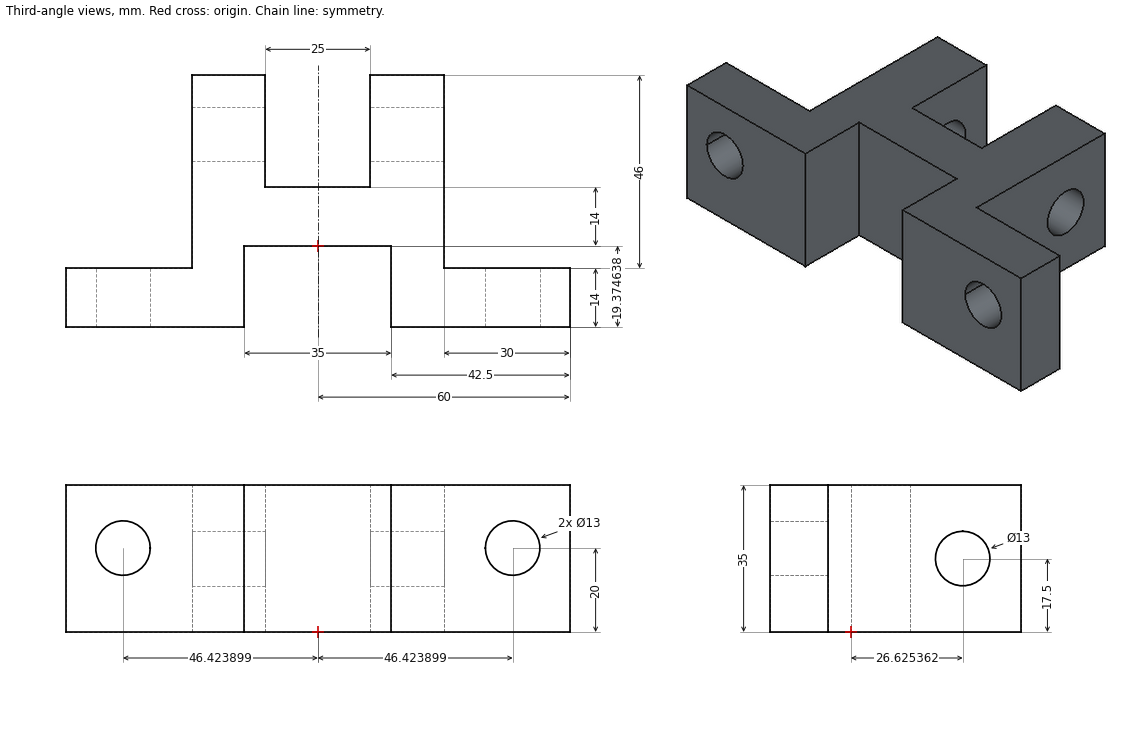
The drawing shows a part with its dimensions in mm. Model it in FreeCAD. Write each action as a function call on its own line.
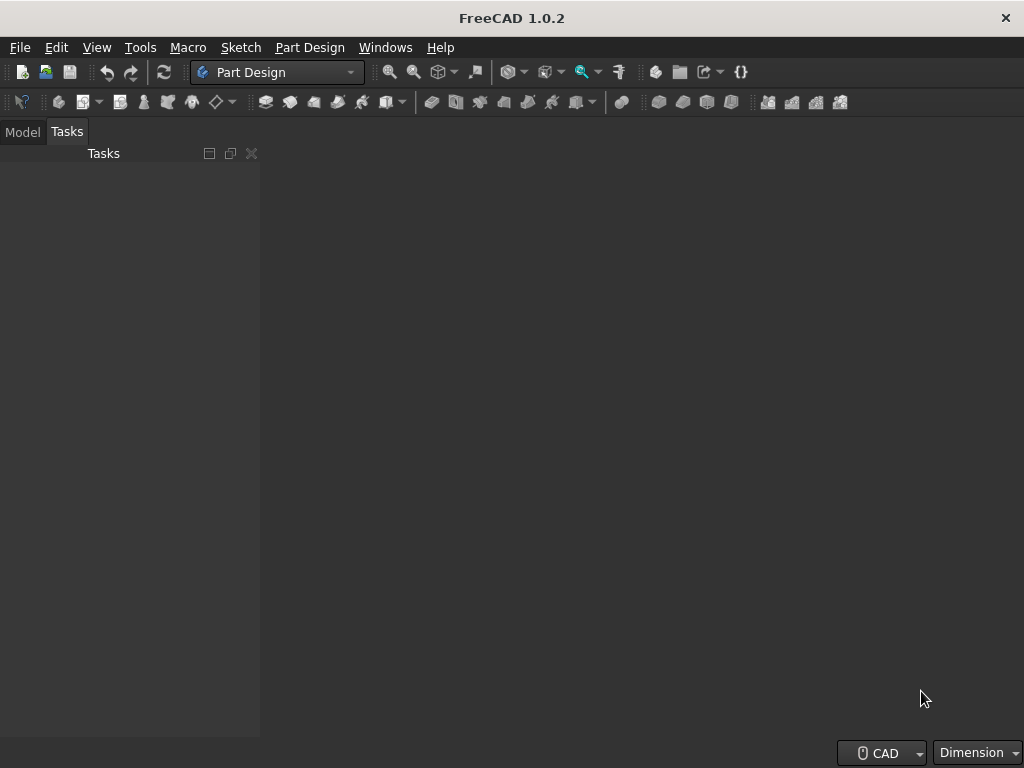
click(22, 72)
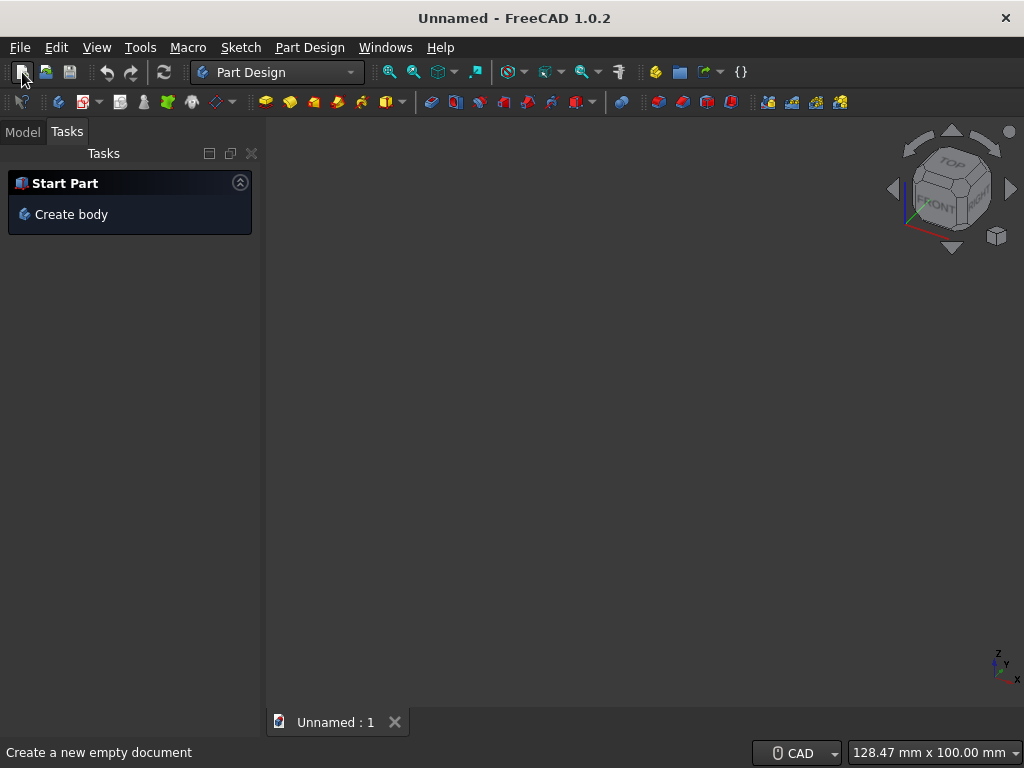
click(84, 102)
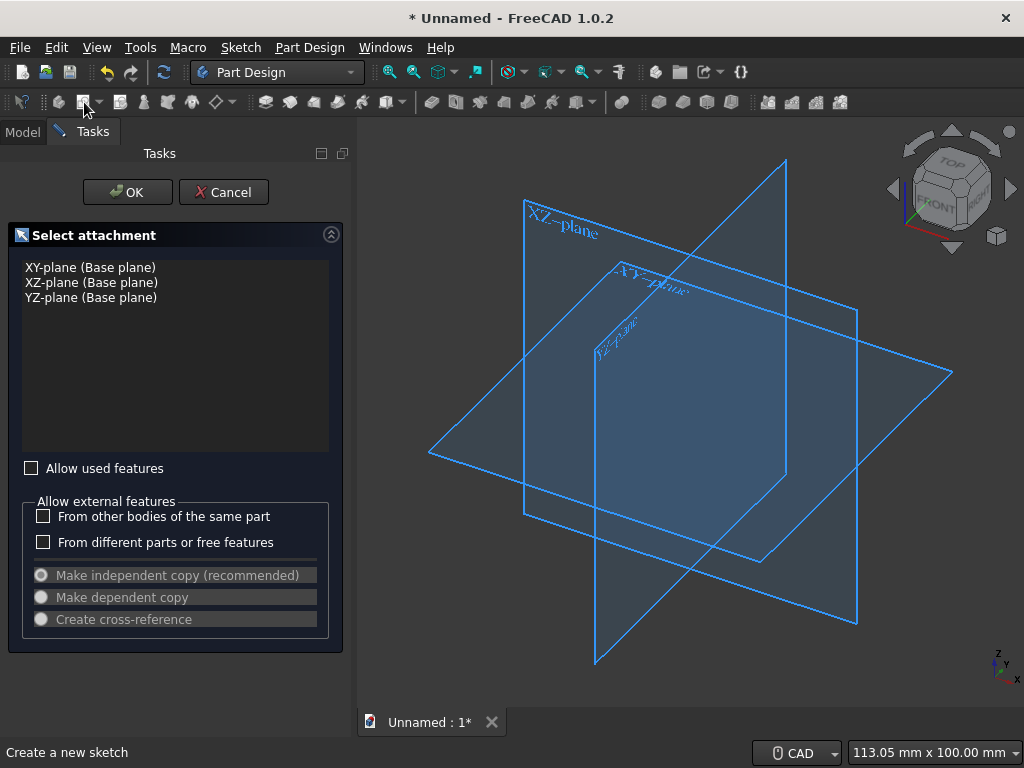
click(82, 268)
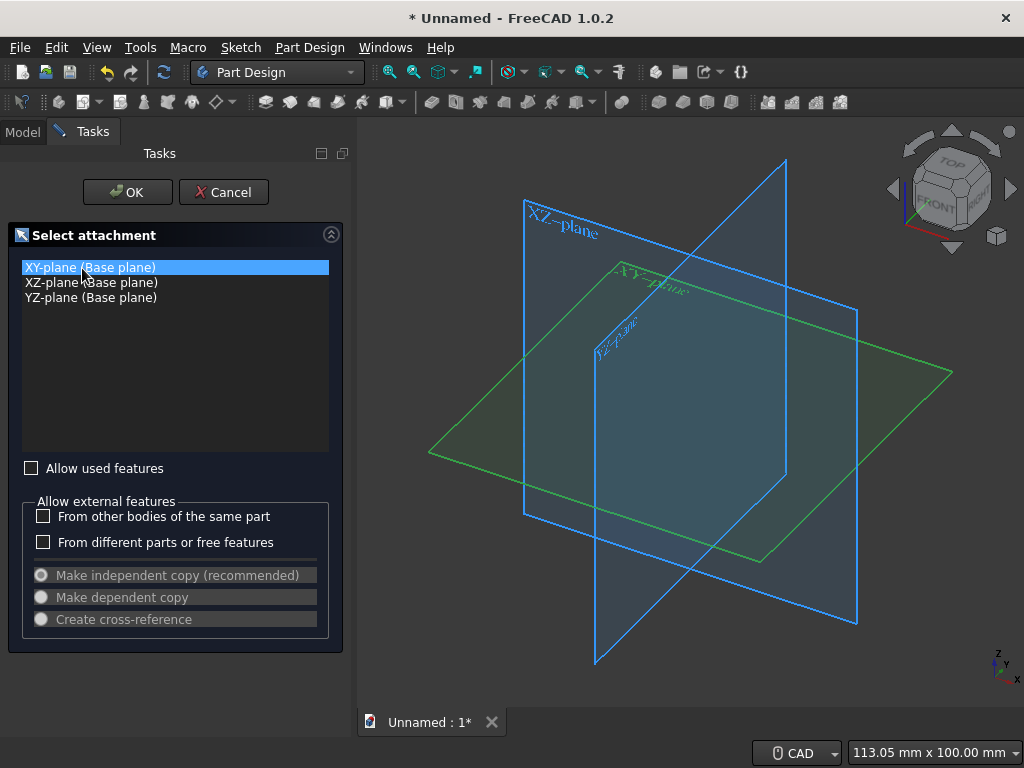
click(128, 192)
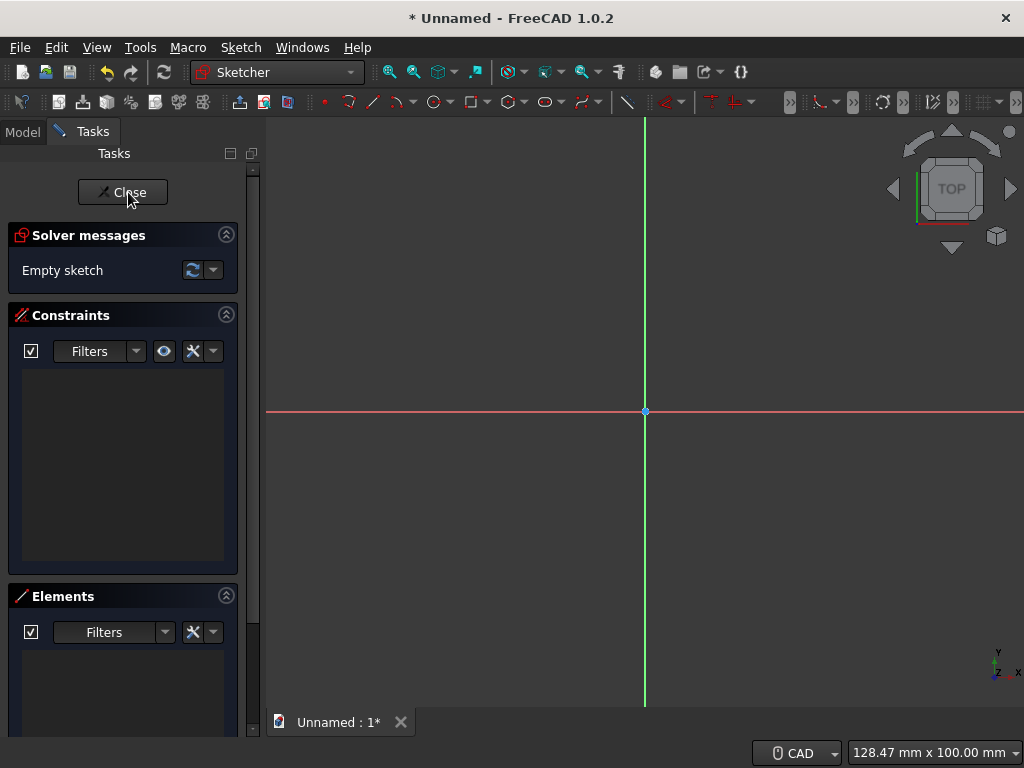
scroll(493, 488, down, 3)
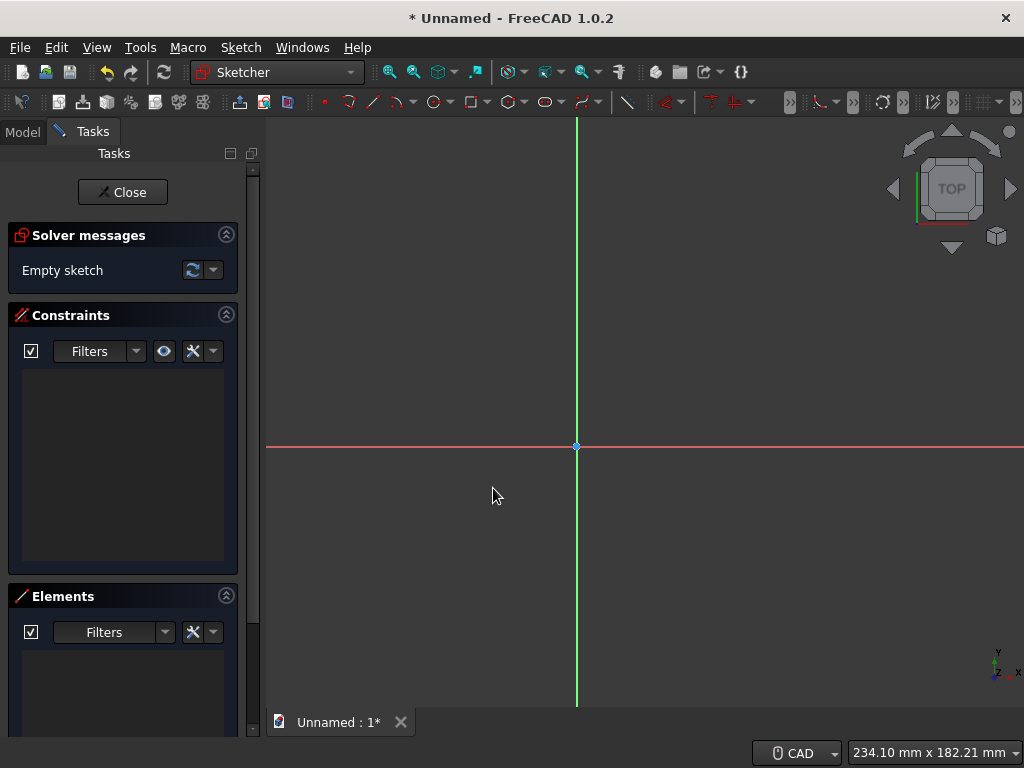
click(350, 102)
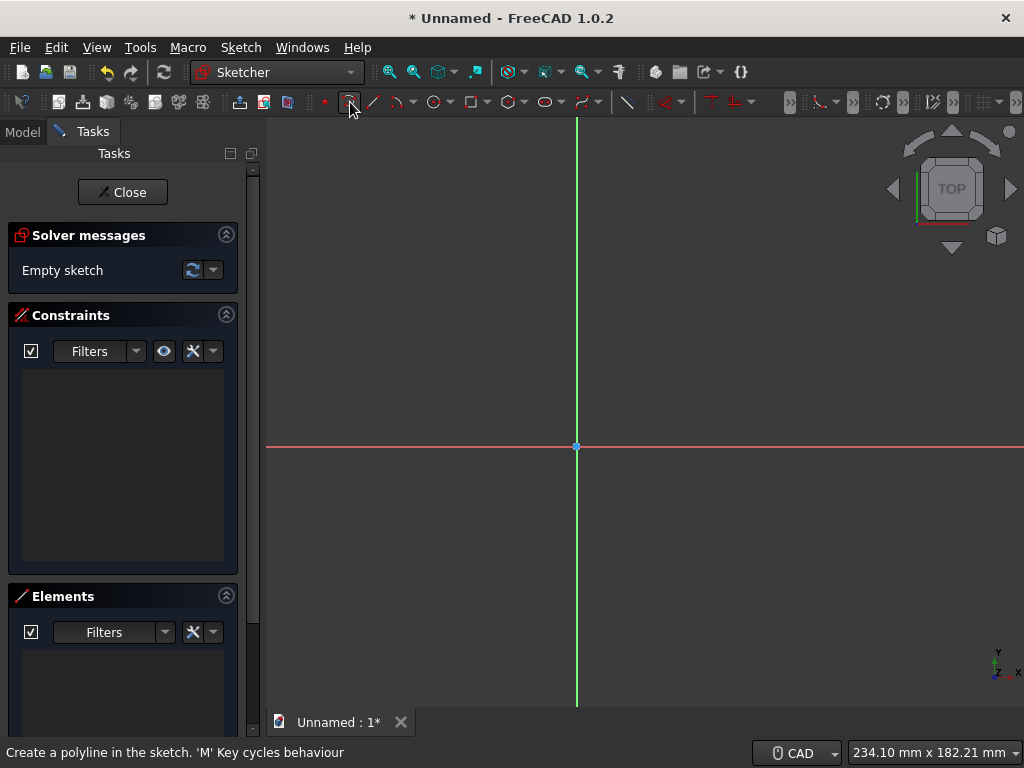
click(633, 447)
click(633, 509)
click(771, 509)
click(771, 464)
click(674, 464)
click(674, 315)
click(617, 315)
click(617, 401)
click(536, 401)
click(536, 315)
click(479, 315)
click(479, 464)
click(382, 464)
click(382, 509)
click(520, 509)
click(520, 438)
click(633, 447)
key(Escape)
key(Escape)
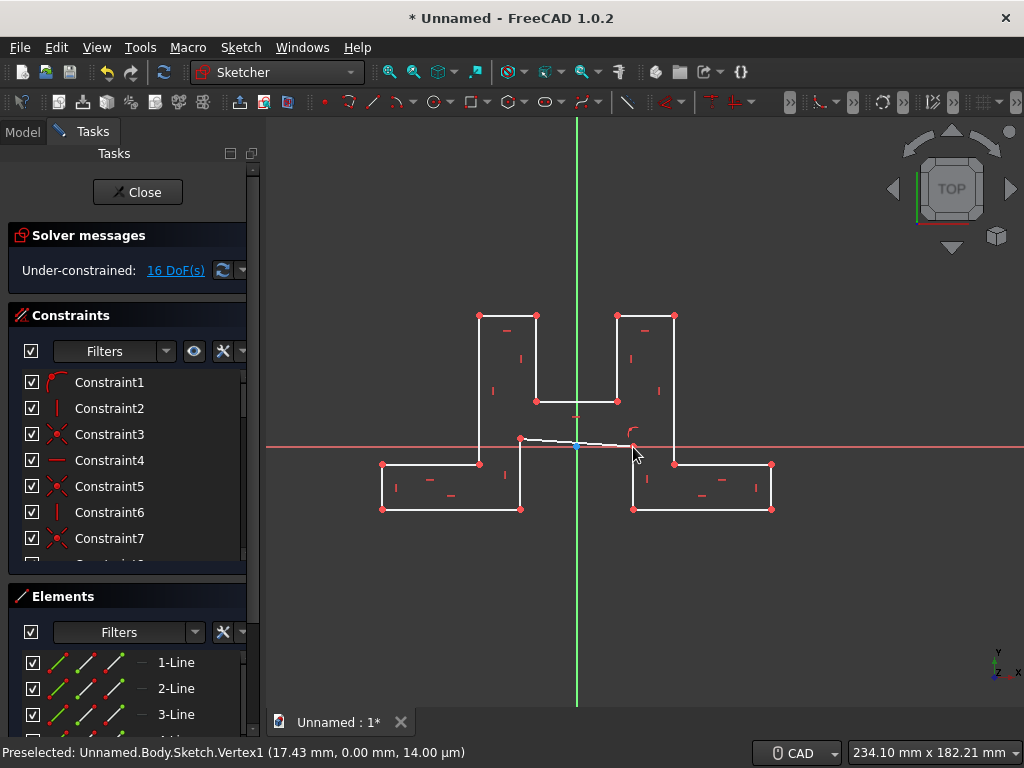
click(599, 444)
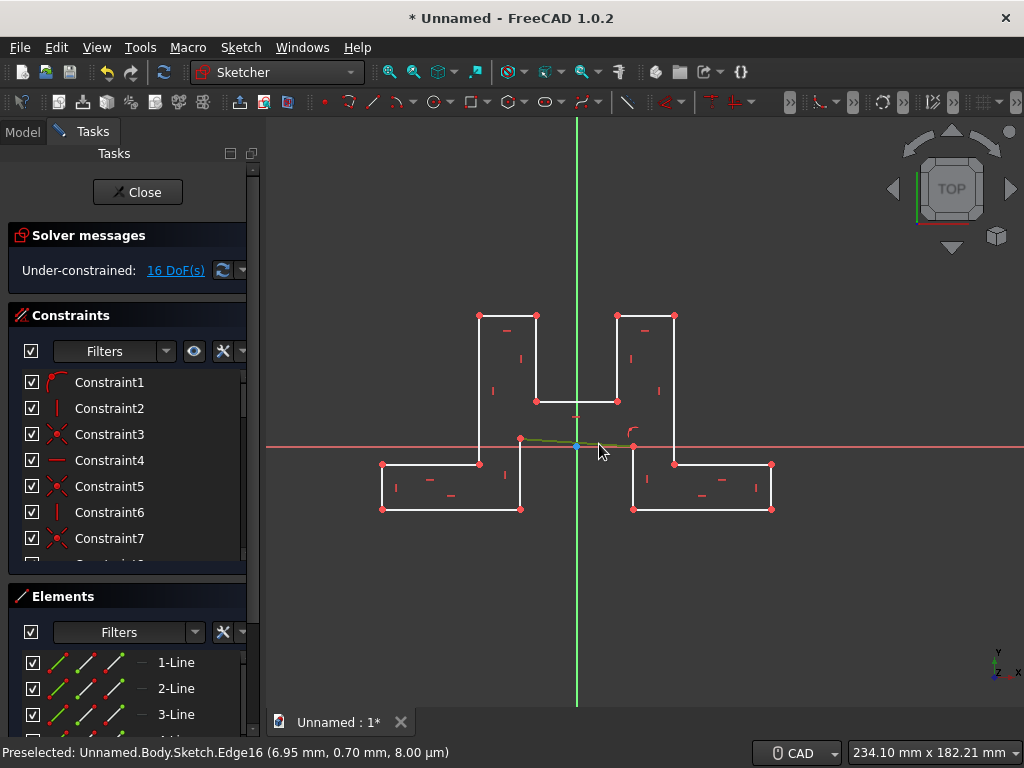
click(754, 102)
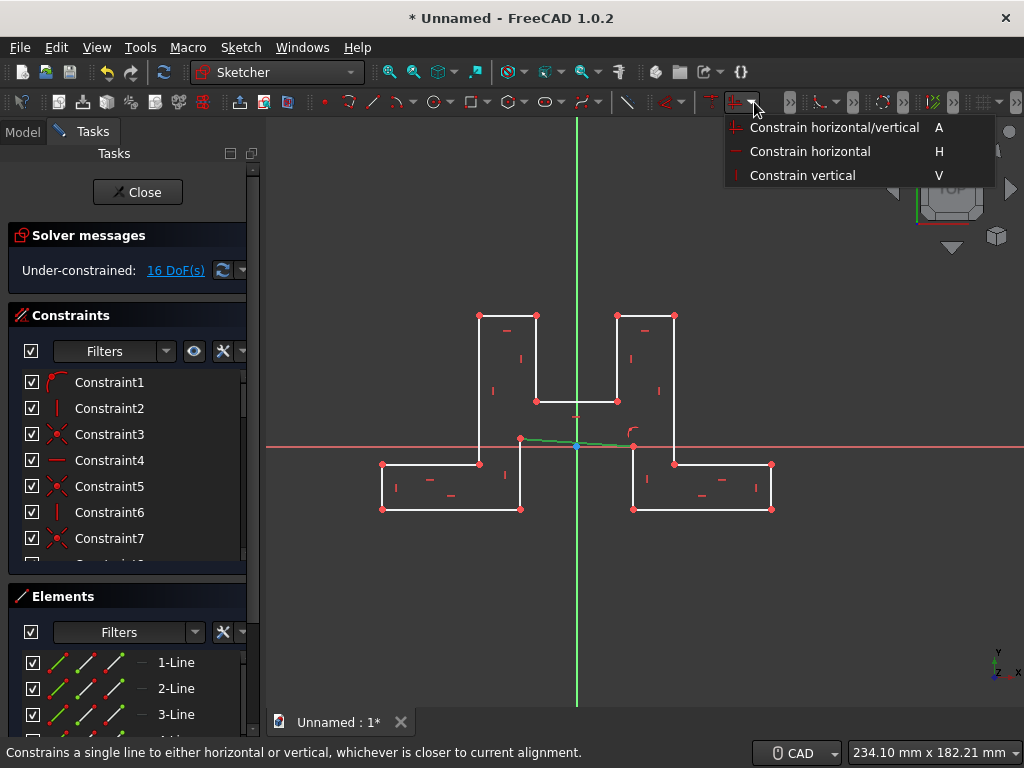
click(860, 151)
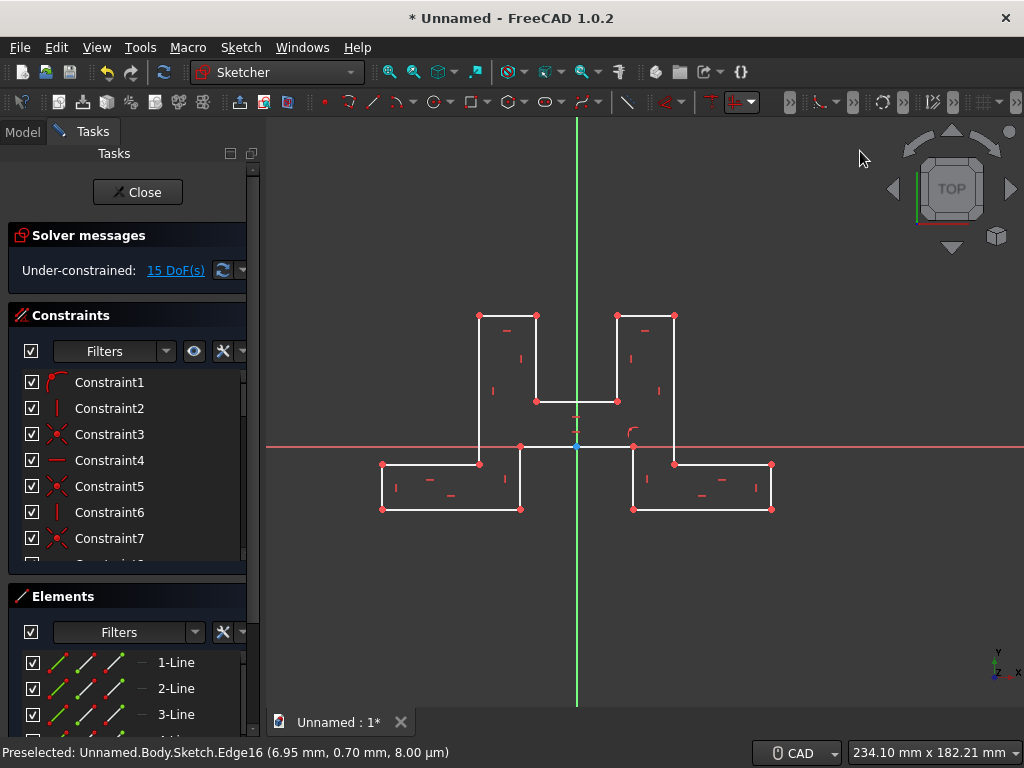
click(617, 316)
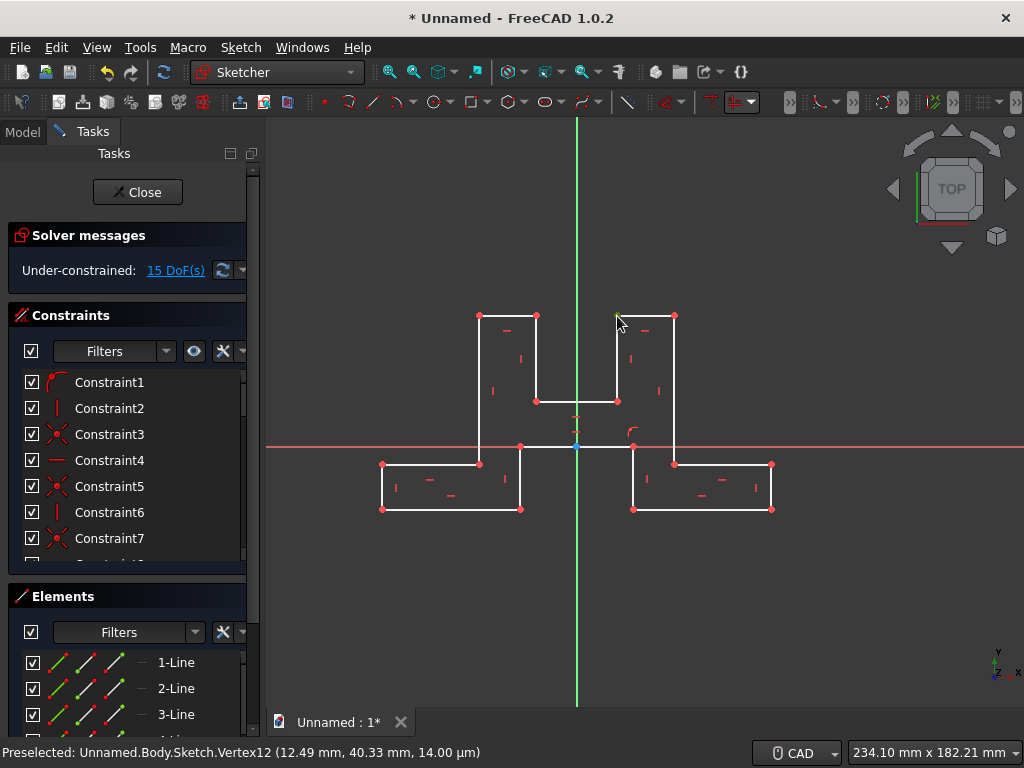
click(536, 316)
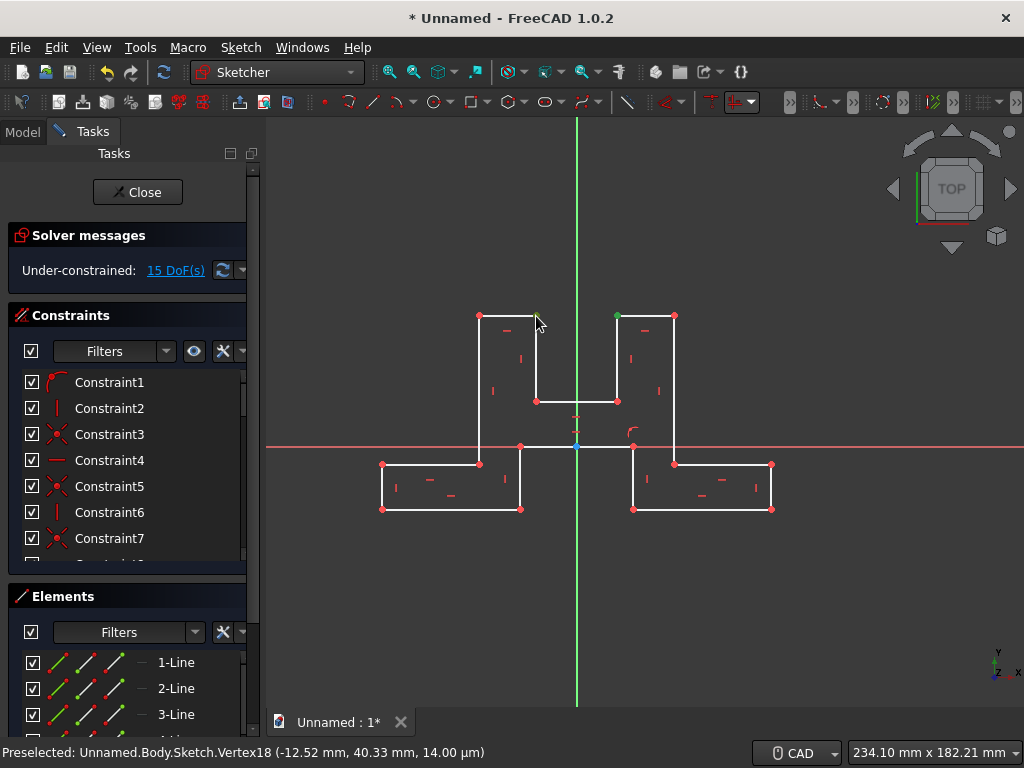
click(577, 641)